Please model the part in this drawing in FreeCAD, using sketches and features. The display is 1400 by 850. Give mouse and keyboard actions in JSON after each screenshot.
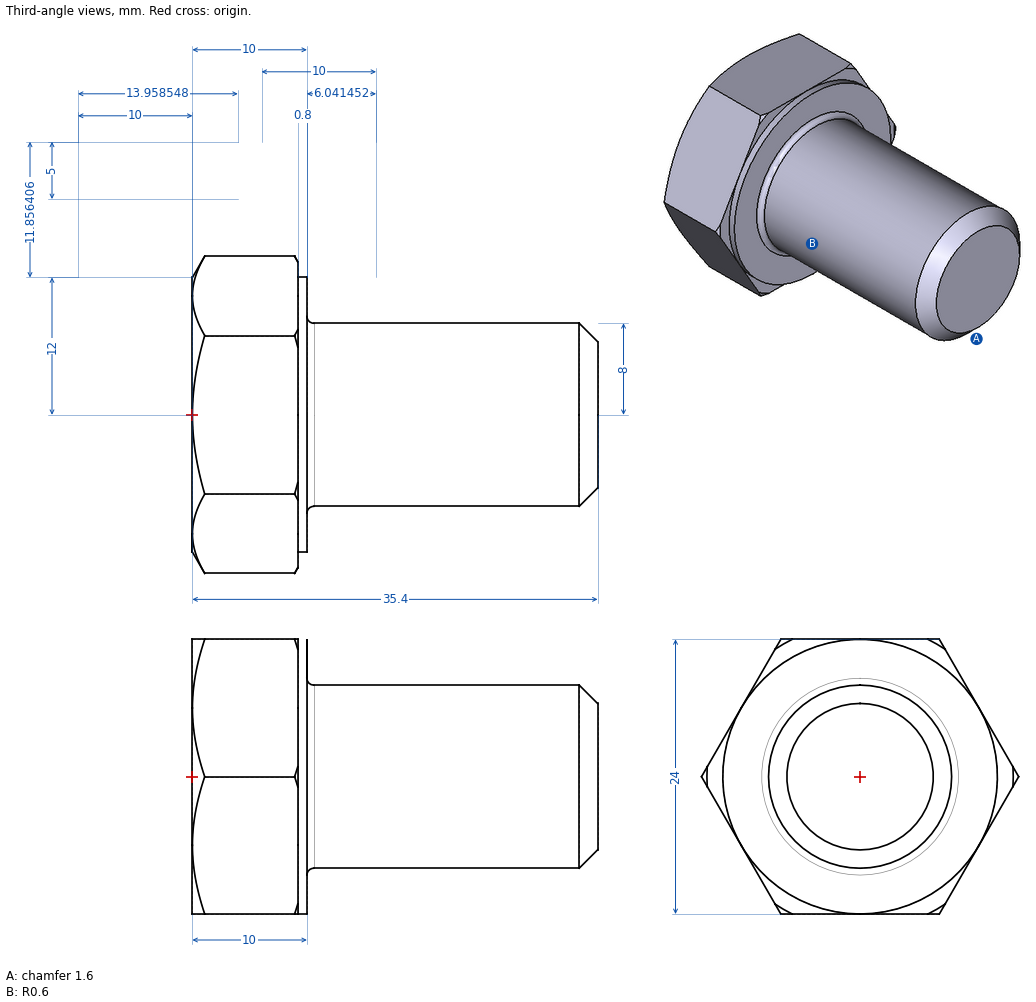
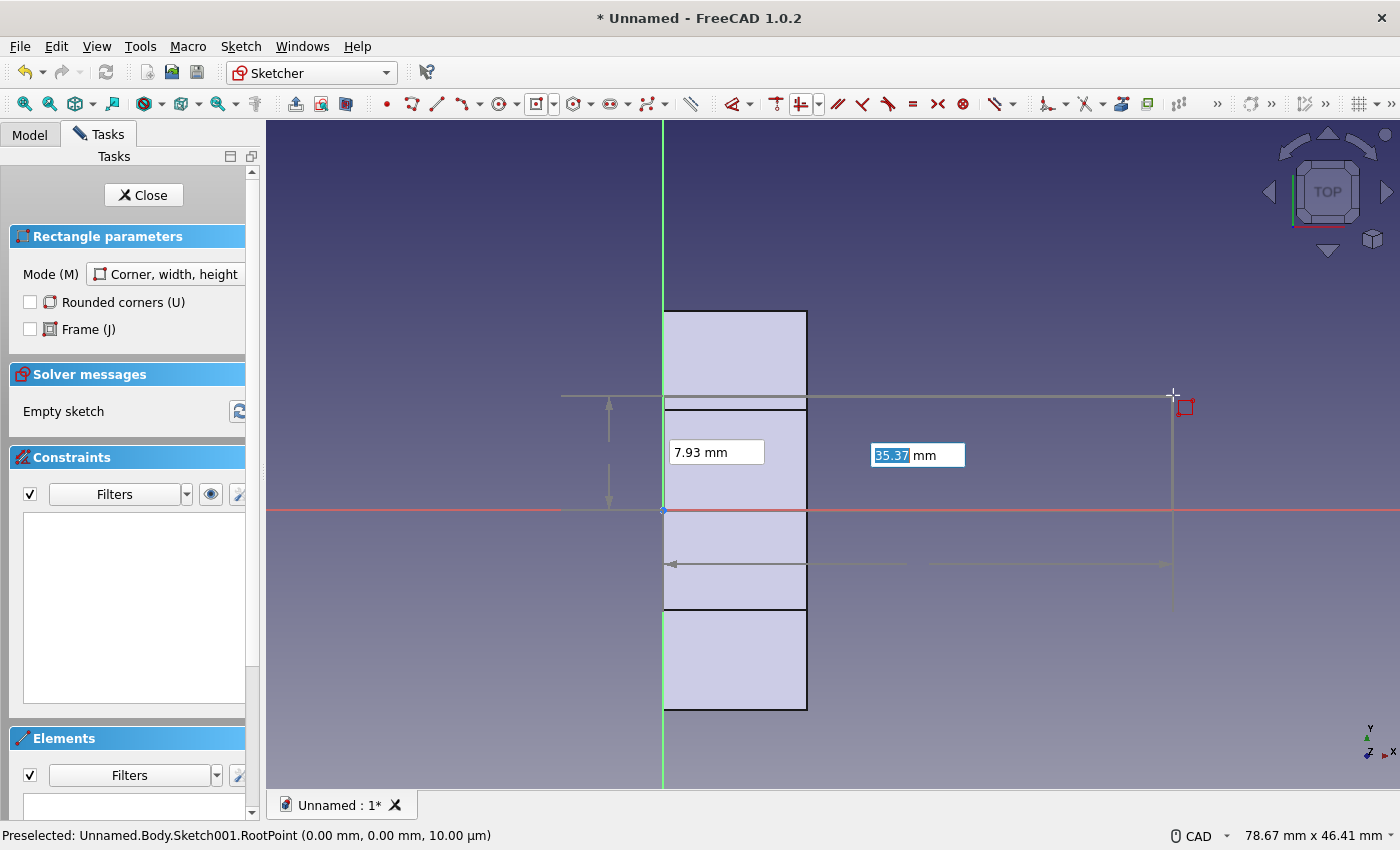
{"action": "type", "text": "35.4"}
{"action": "key", "text": "Tab"}
{"action": "type", "text": "8"}
{"action": "key", "text": "Return"}
{"action": "key", "text": "Escape"}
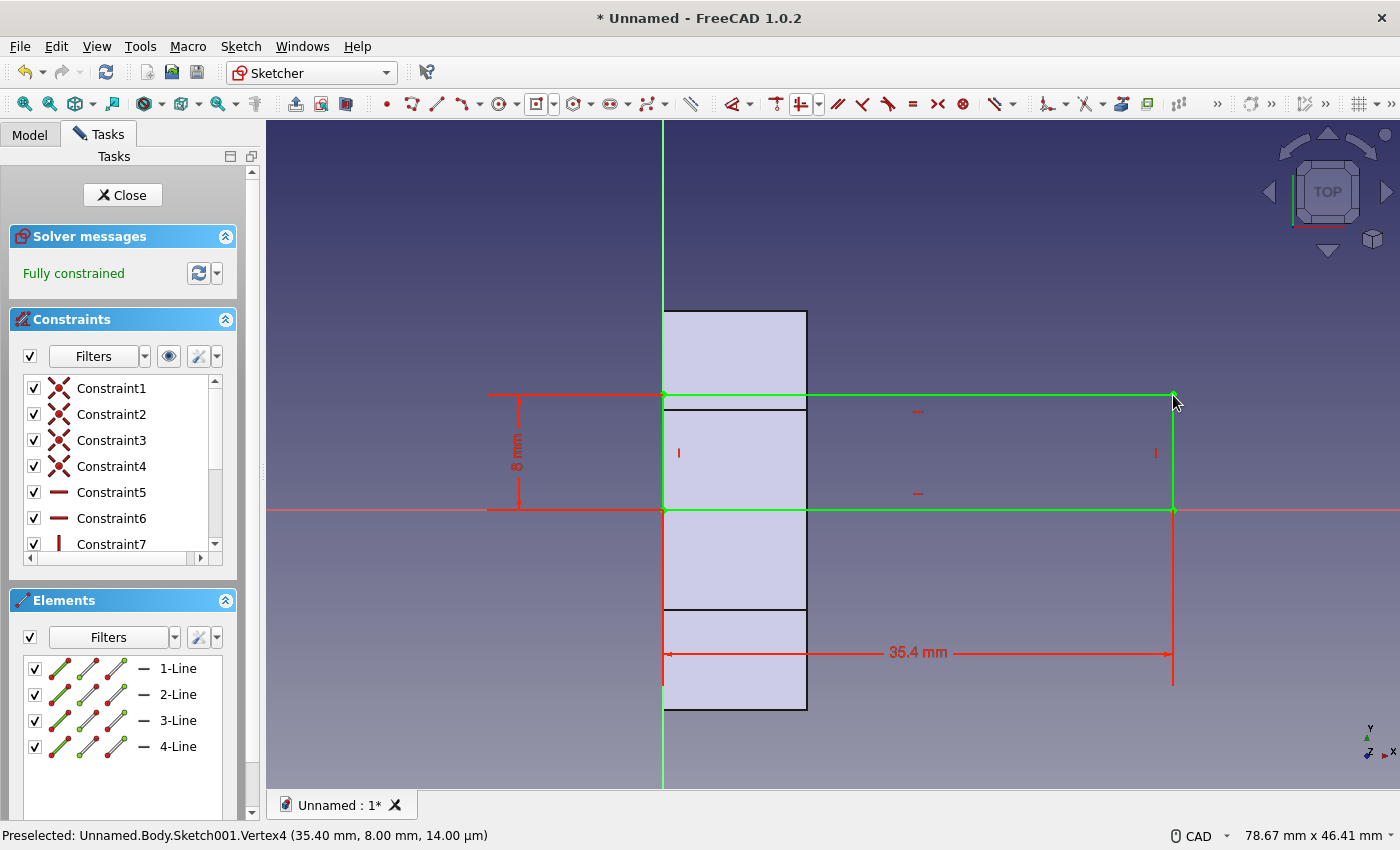
{"action": "left_click", "coordinate": [123, 195]}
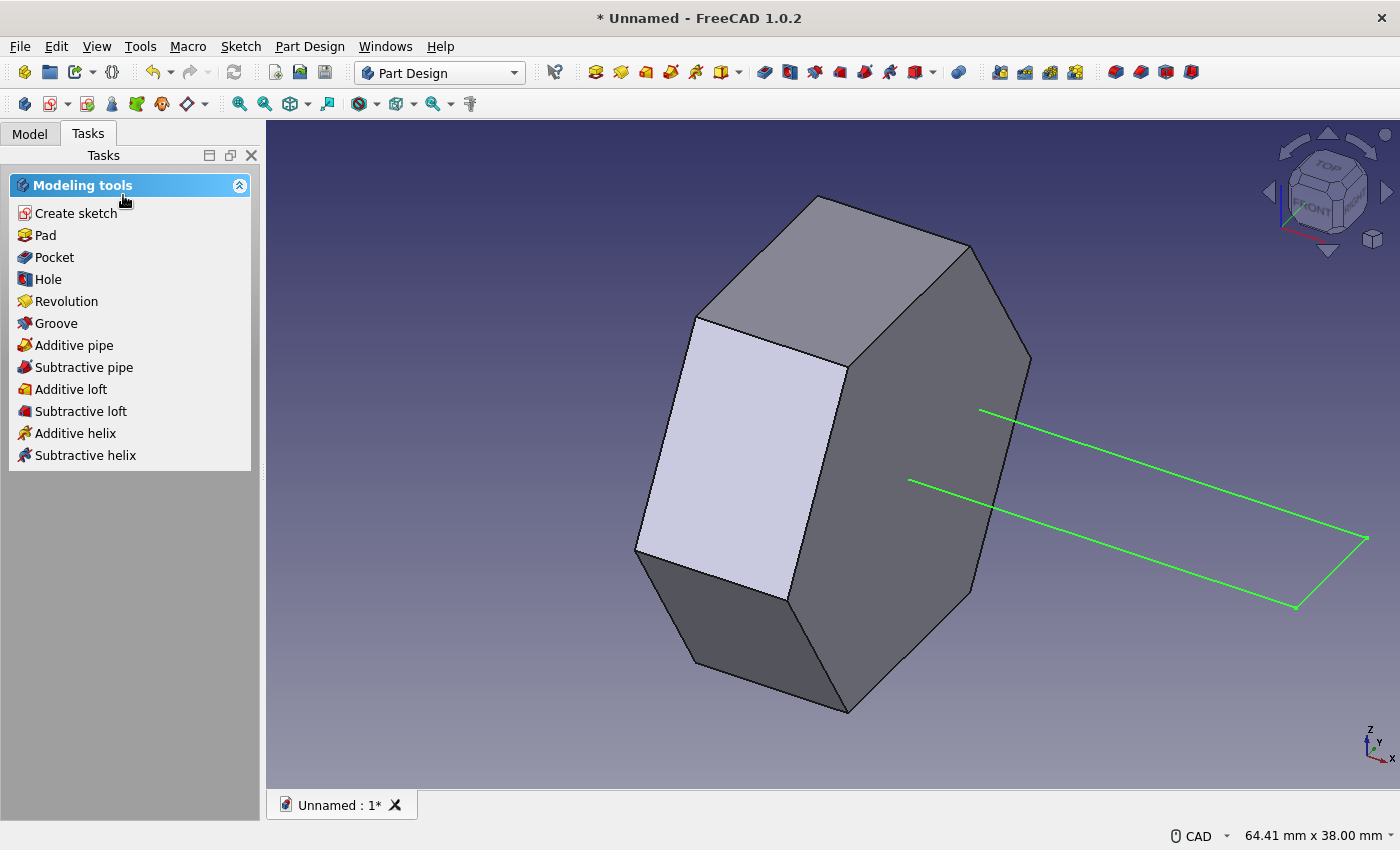
{"action": "left_click", "coordinate": [621, 72]}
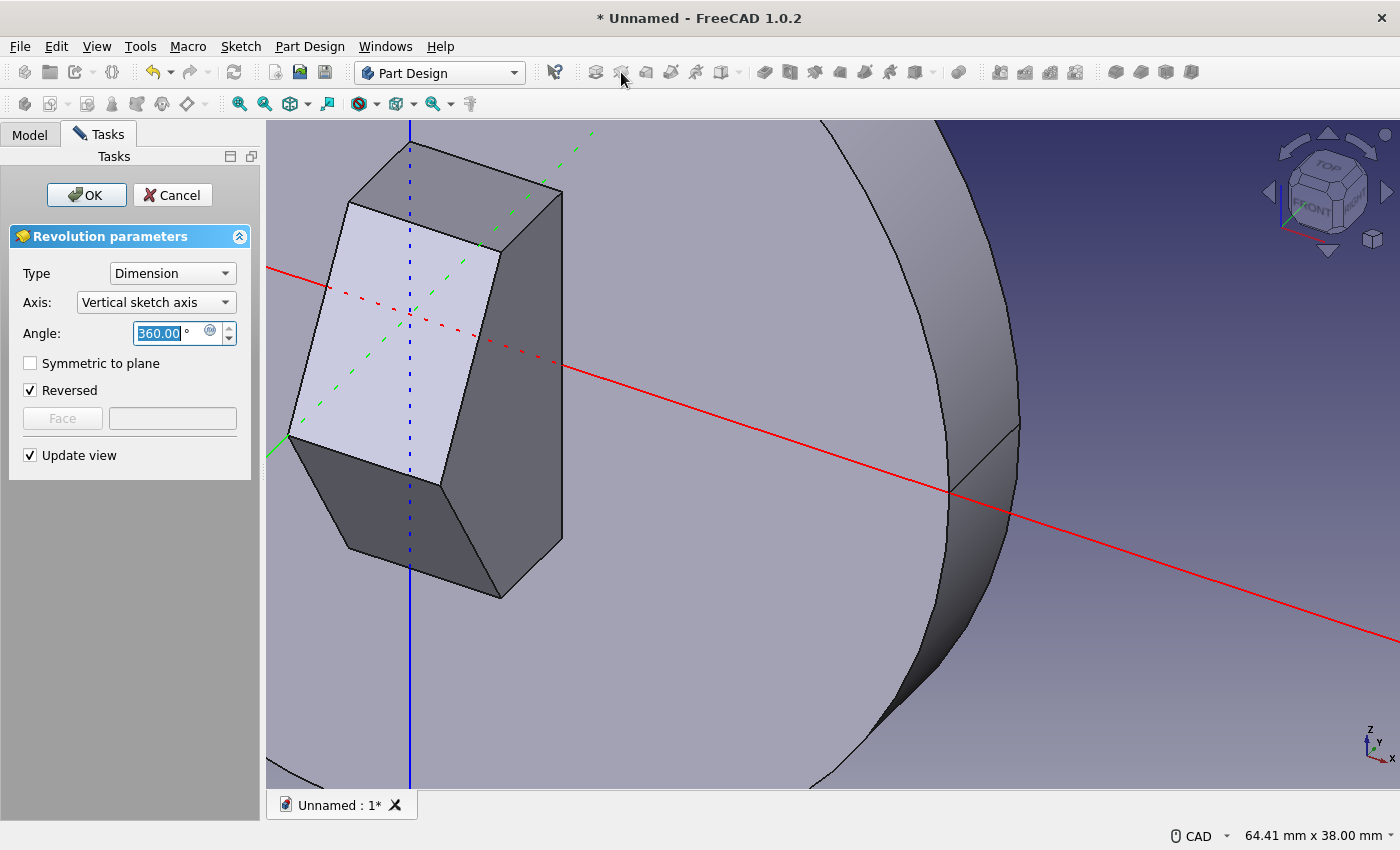
{"action": "left_click", "coordinate": [157, 302]}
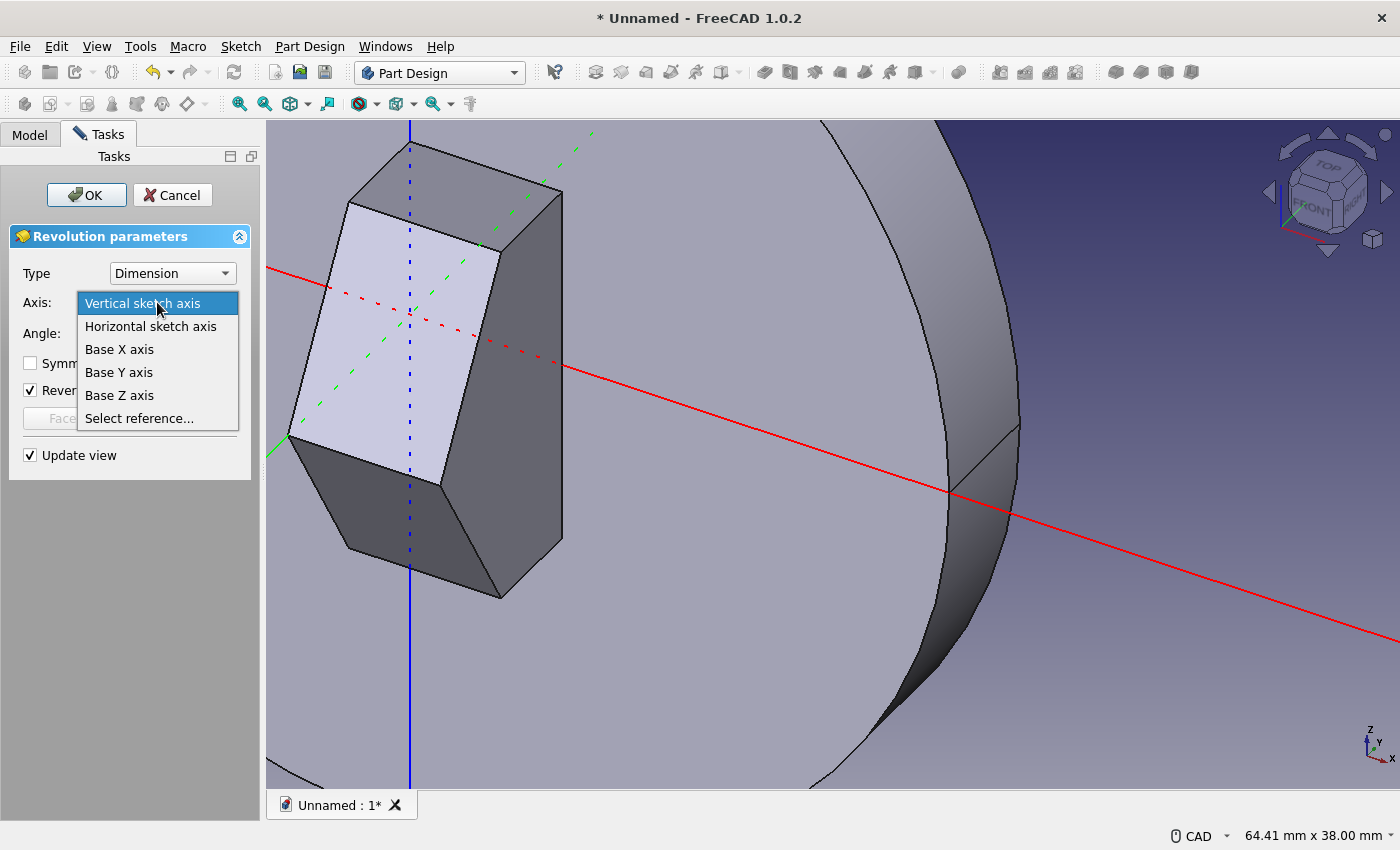
{"action": "left_click", "coordinate": [156, 326]}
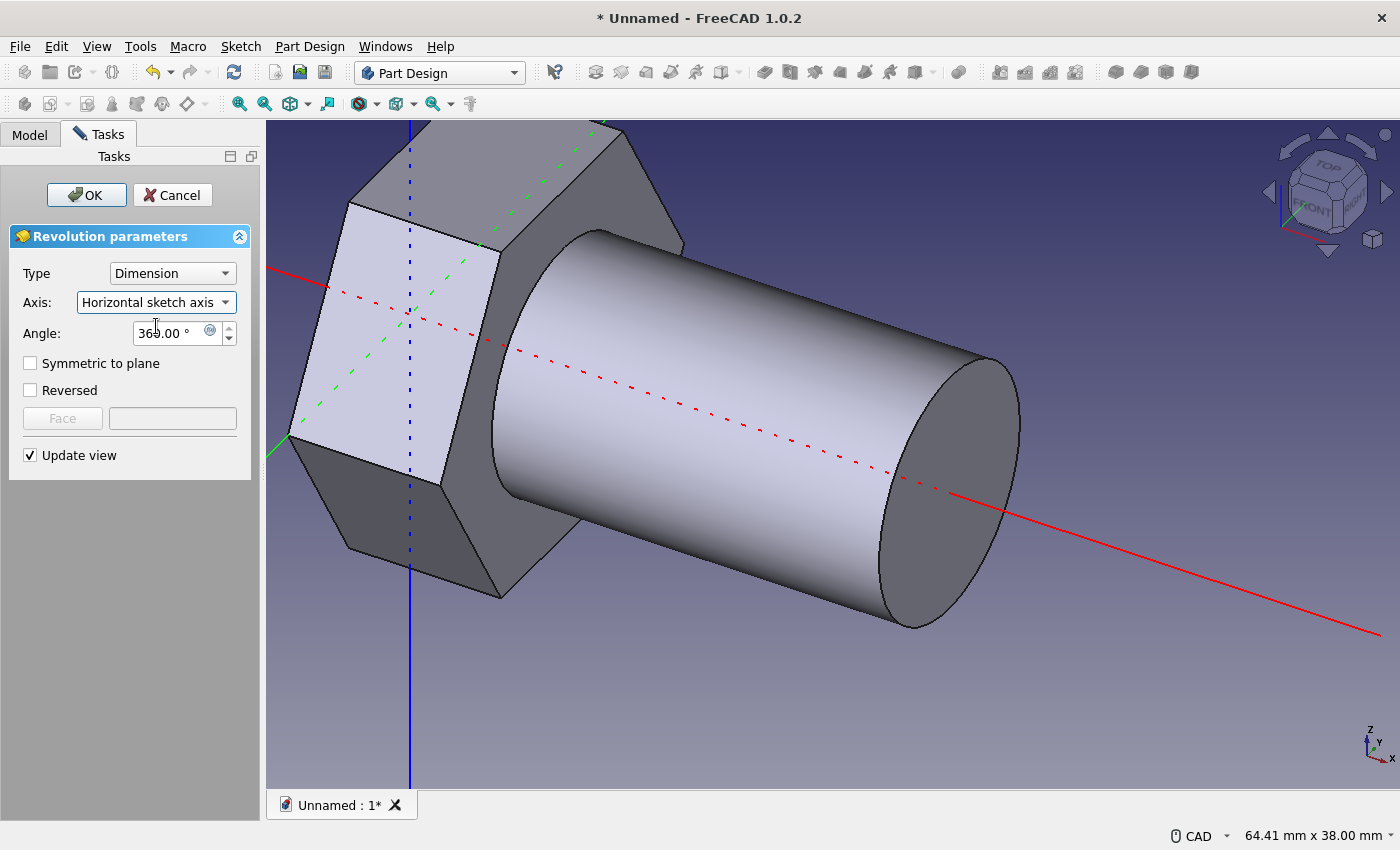
{"action": "left_click", "coordinate": [87, 195]}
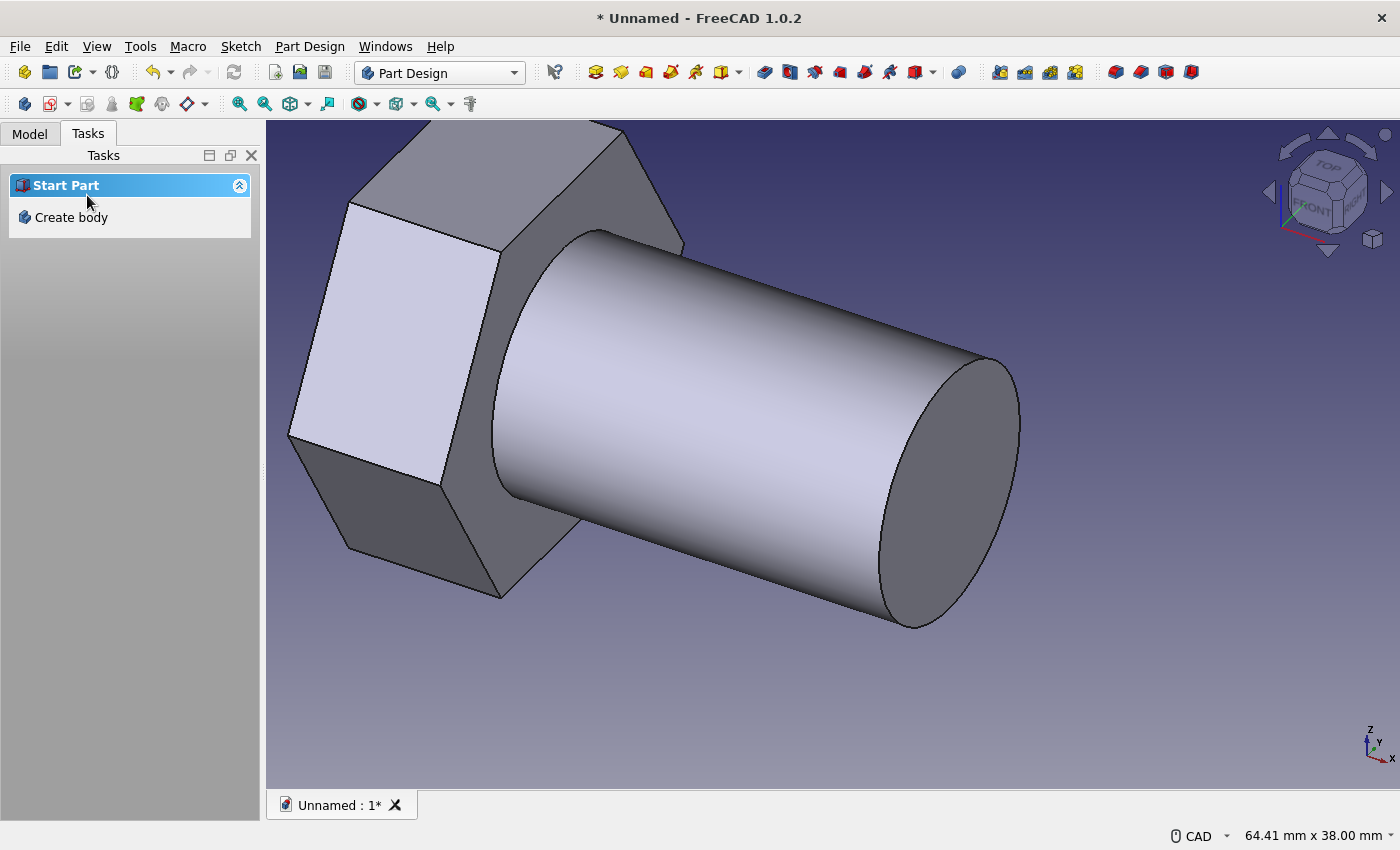
{"action": "left_click", "coordinate": [240, 104]}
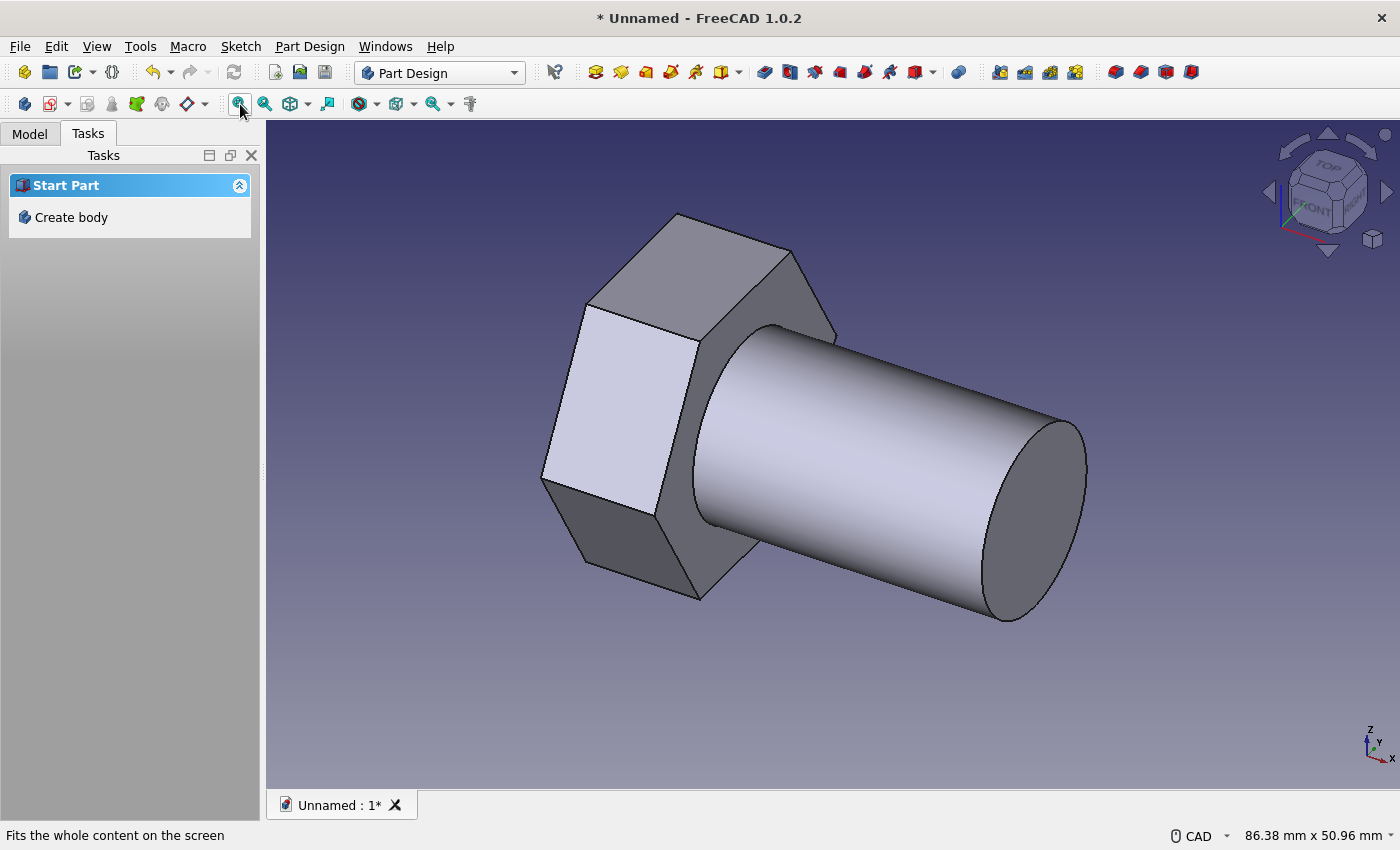
{"action": "left_click", "coordinate": [50, 104]}